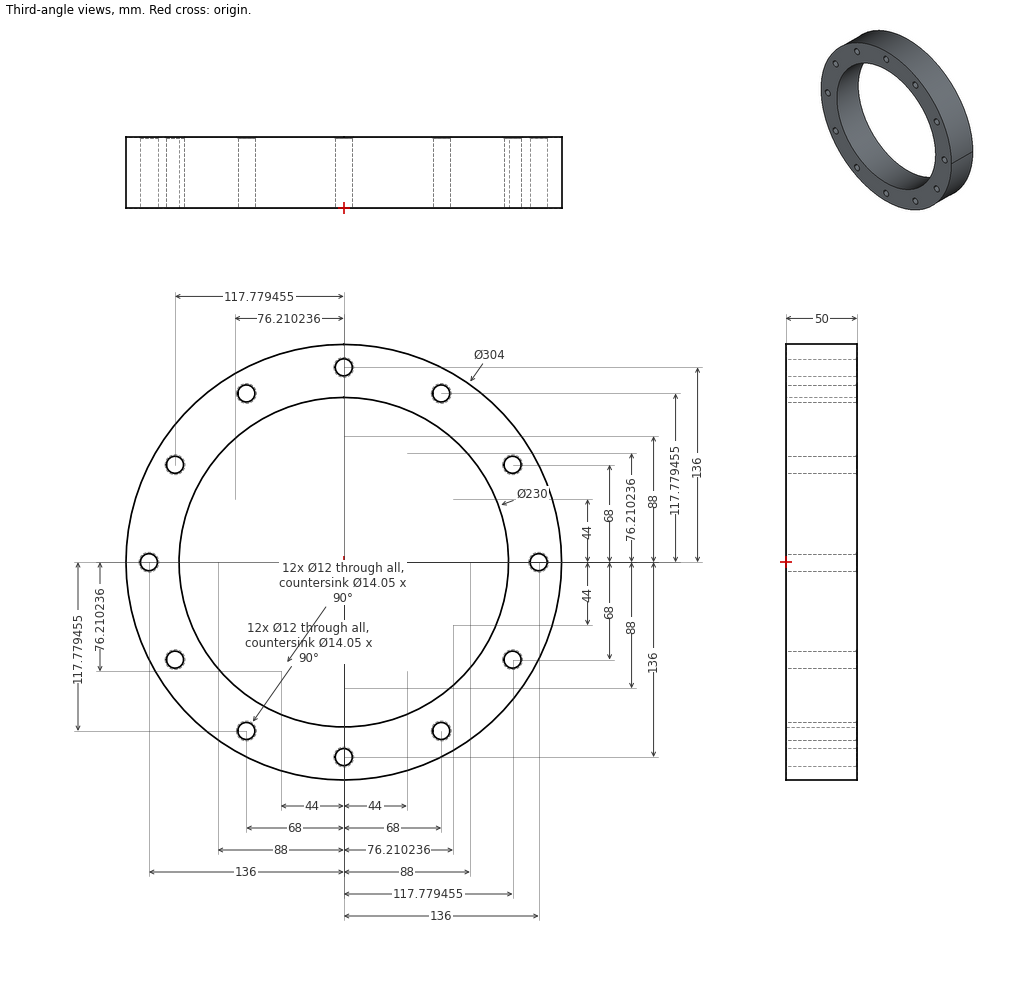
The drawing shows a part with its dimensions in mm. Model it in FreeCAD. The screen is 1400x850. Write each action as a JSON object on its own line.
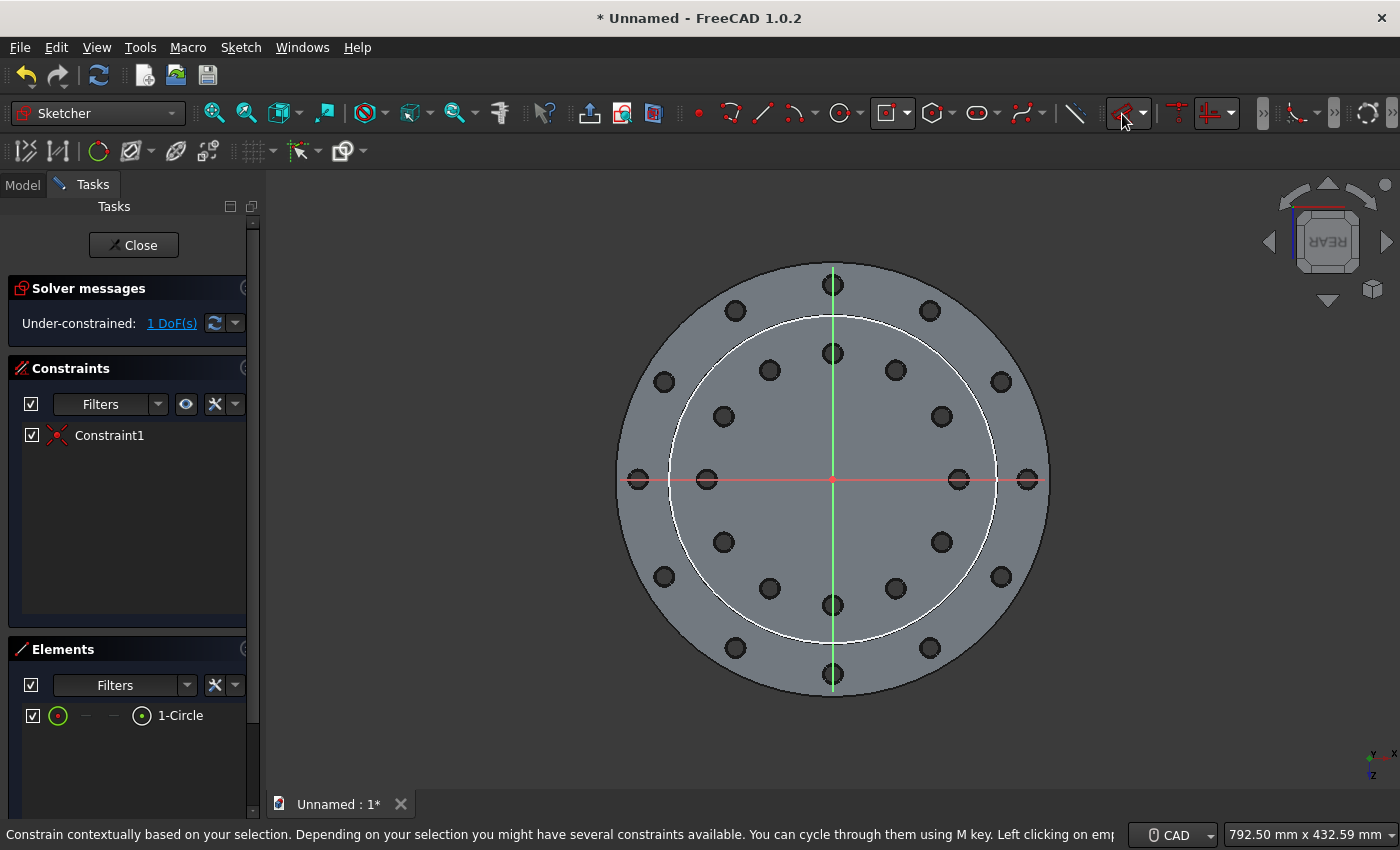
{"action": "left_click", "coordinate": [948, 363]}
{"action": "left_click", "coordinate": [970, 340]}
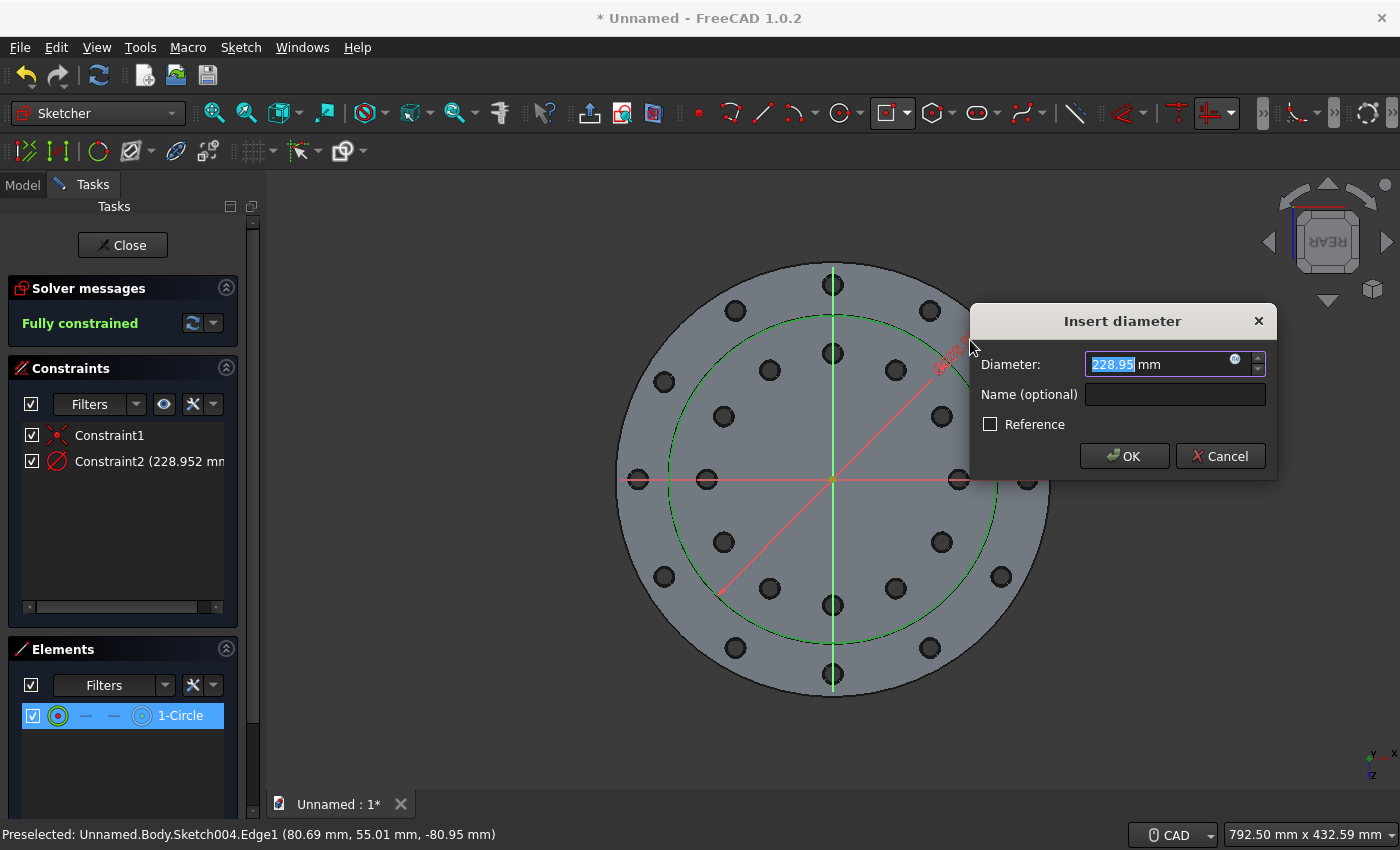
{"action": "type", "text": "230"}
{"action": "key", "text": "Return"}
{"action": "key", "text": "Escape"}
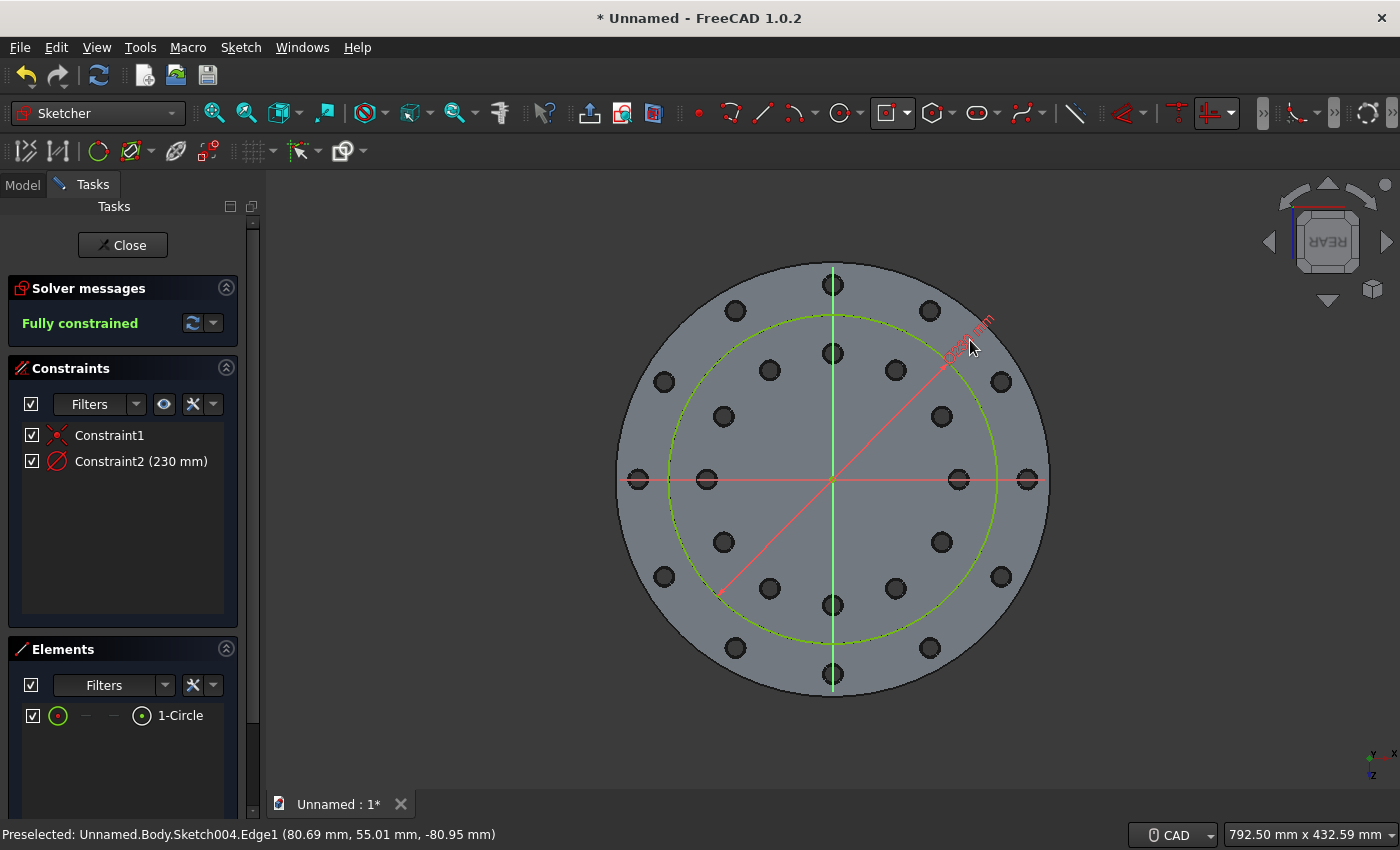
{"action": "left_click", "coordinate": [123, 245]}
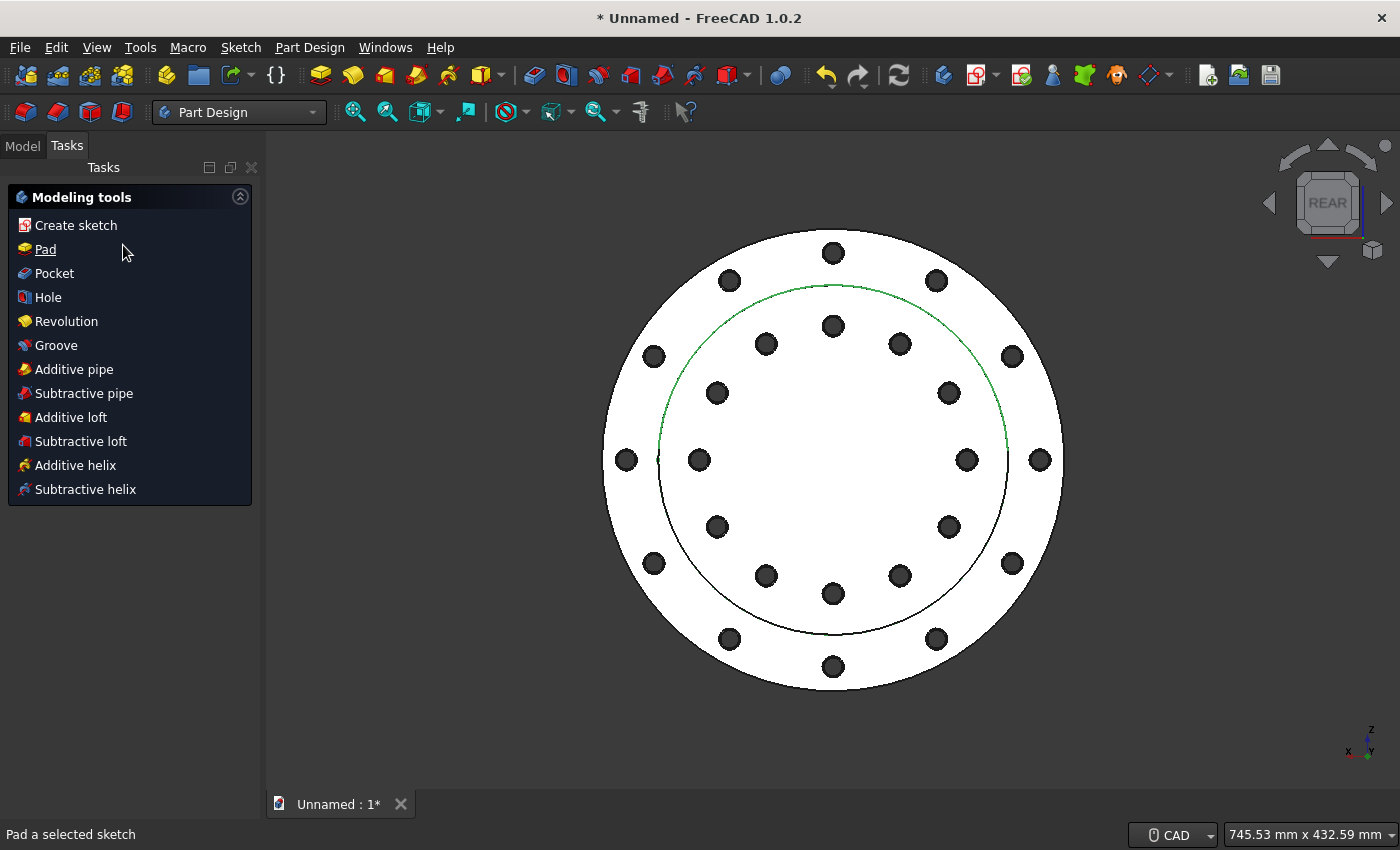
{"action": "left_click", "coordinate": [536, 76]}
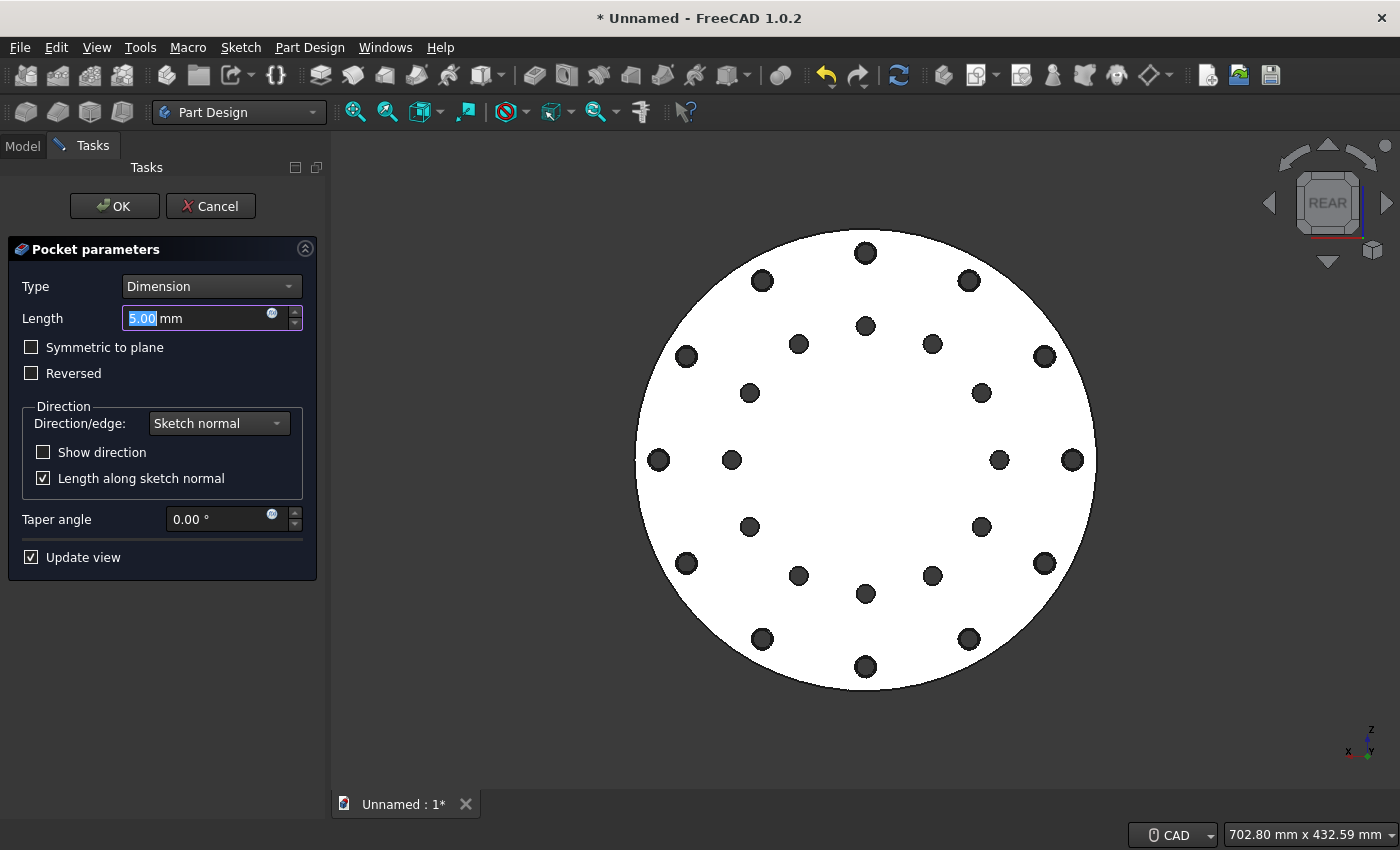
{"action": "left_click", "coordinate": [212, 286]}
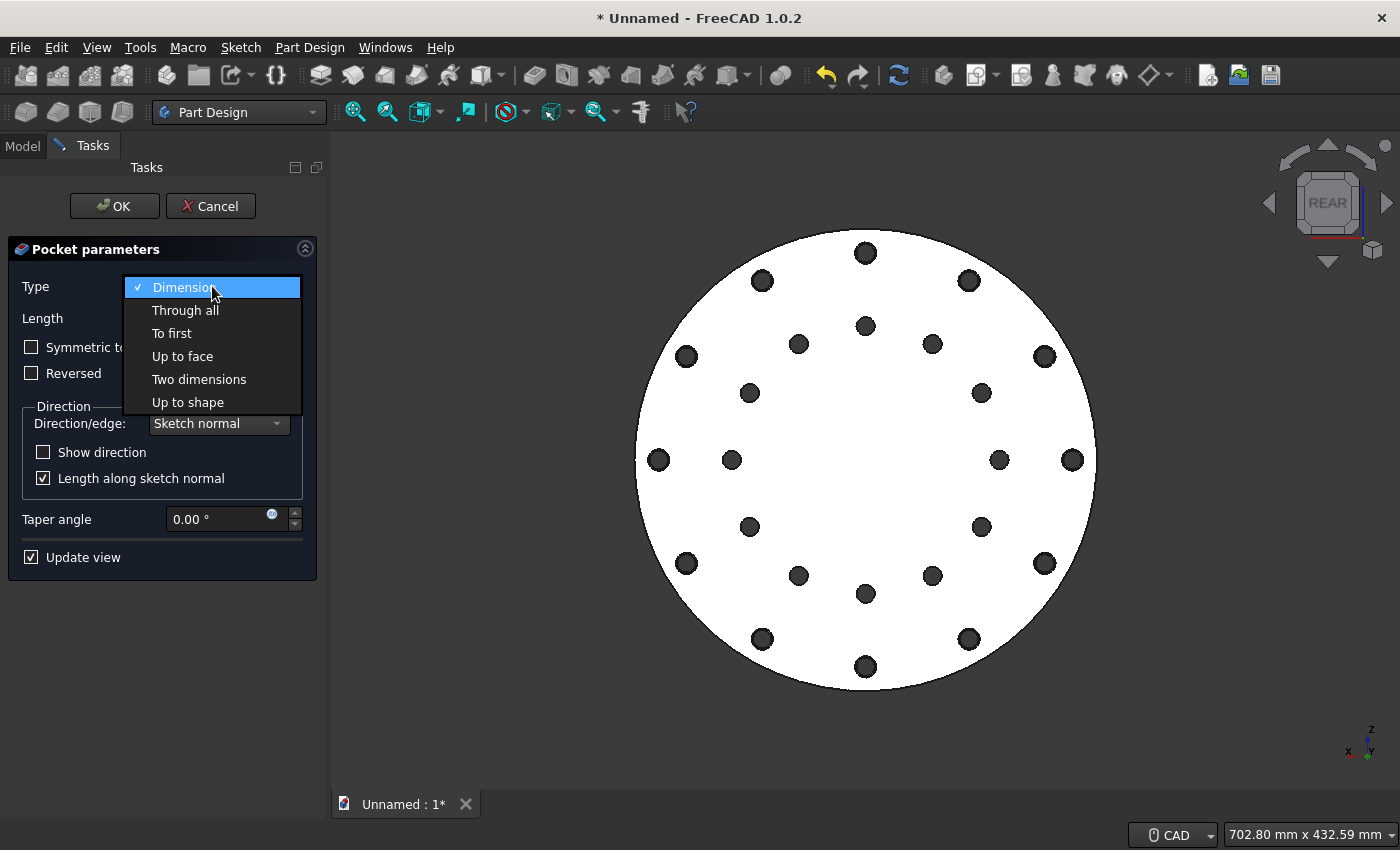
{"action": "left_click", "coordinate": [212, 310]}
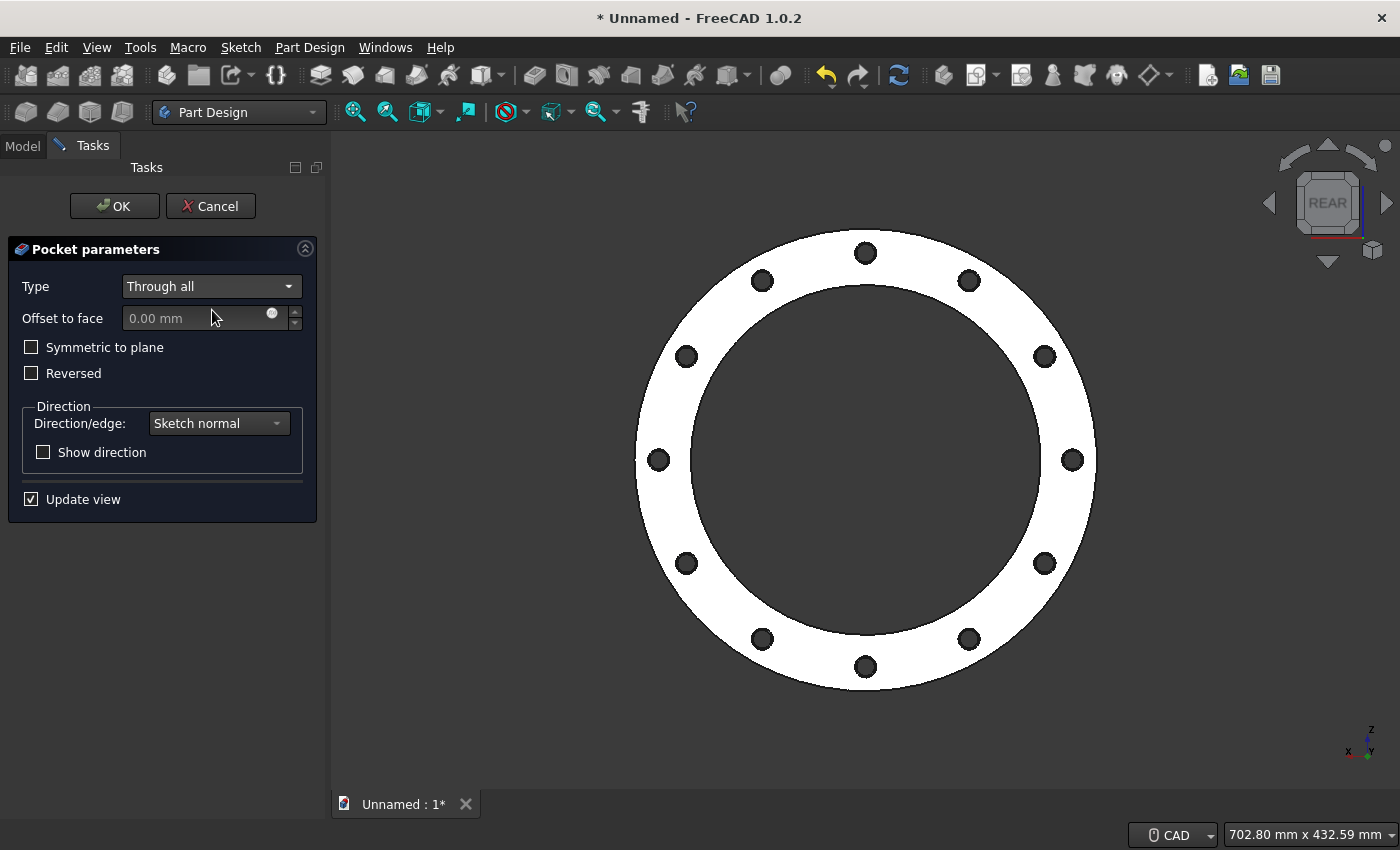
{"action": "left_click", "coordinate": [115, 206]}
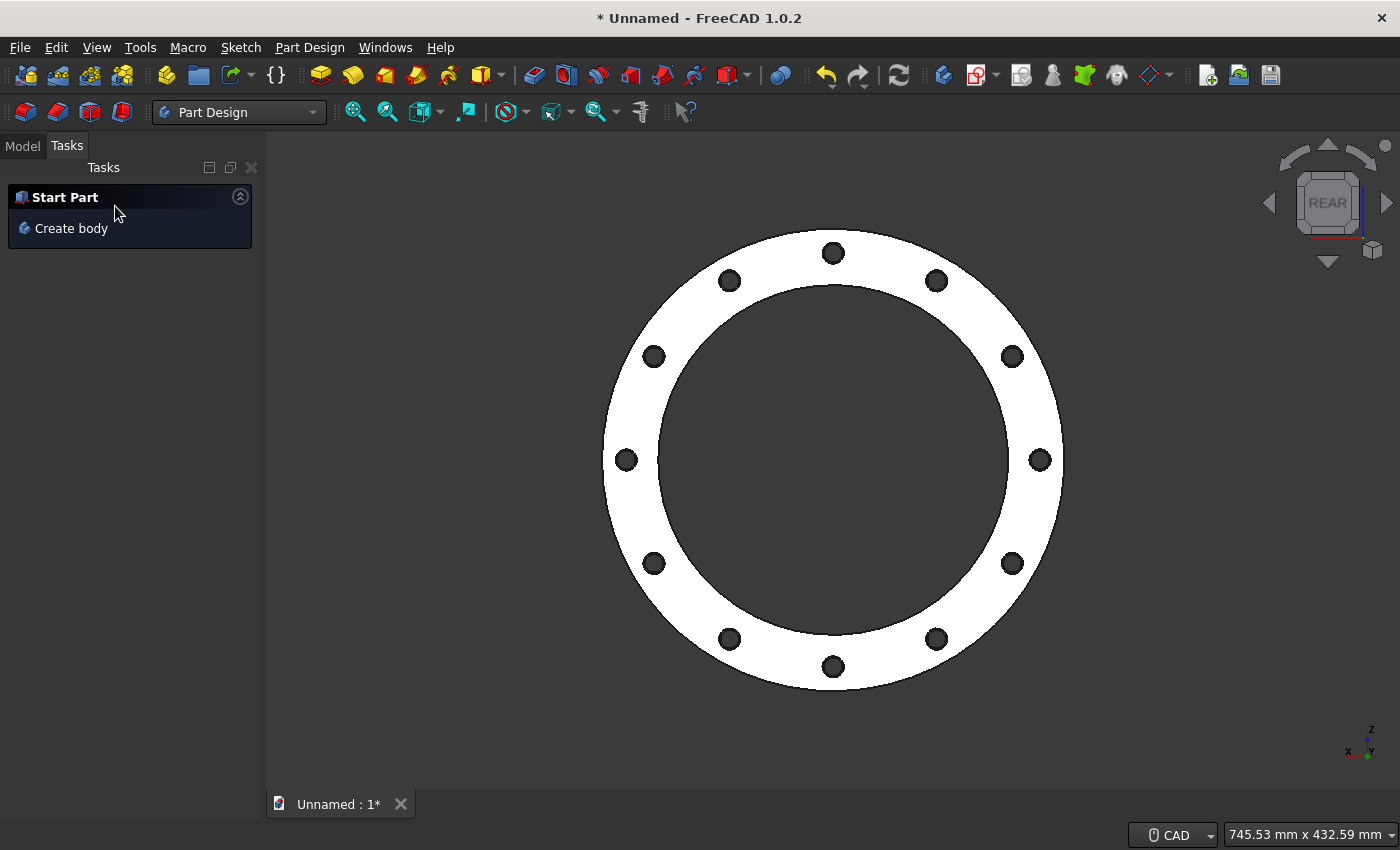
{"action": "key", "text": "0"}